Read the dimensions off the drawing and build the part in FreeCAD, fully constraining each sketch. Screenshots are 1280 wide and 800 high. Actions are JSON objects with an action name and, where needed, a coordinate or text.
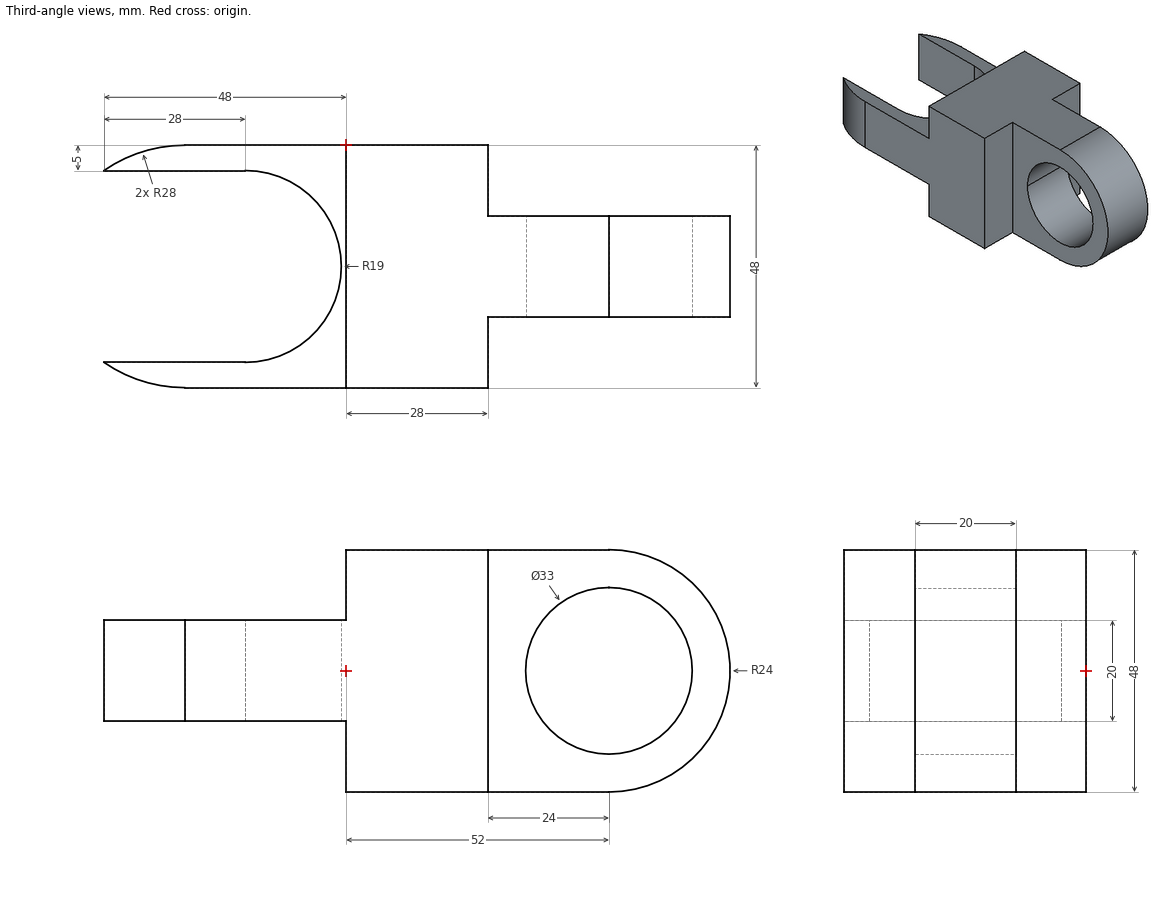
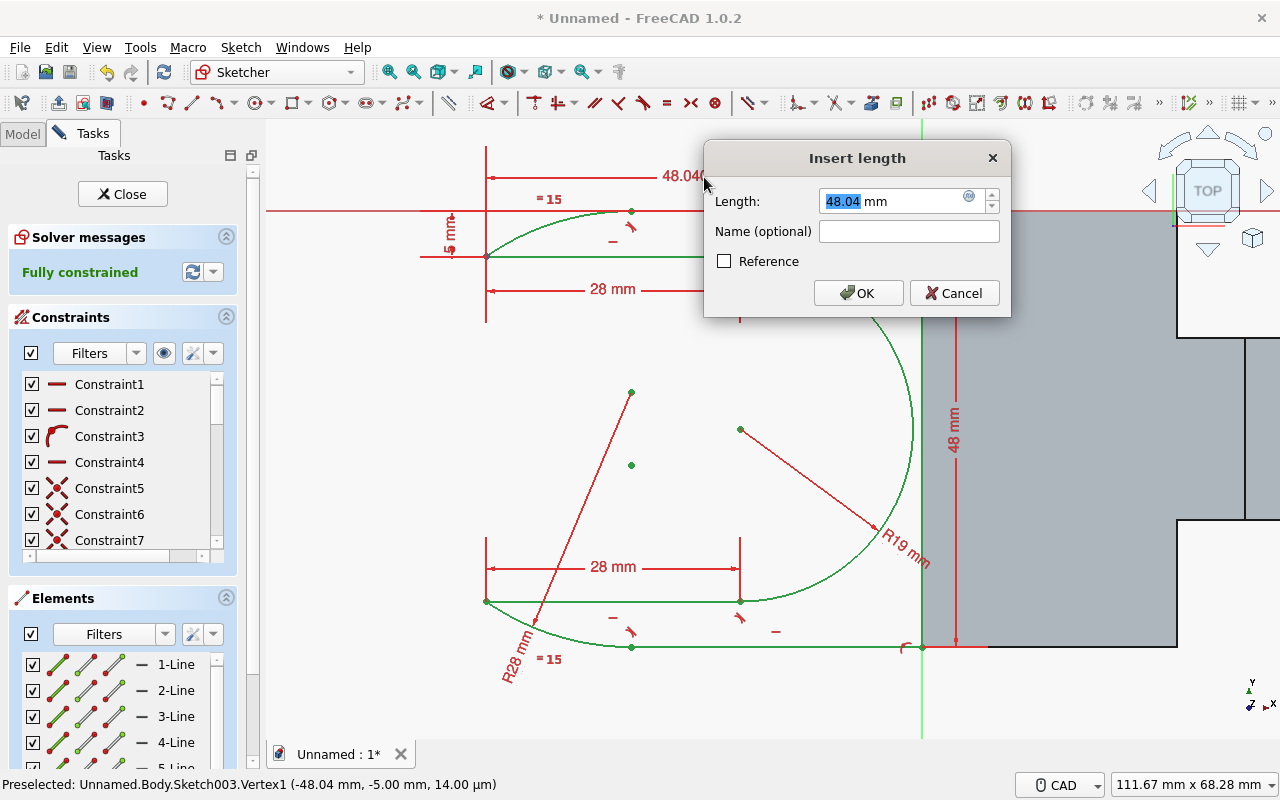
{"action": "type", "text": "48"}
{"action": "key", "text": "Return"}
{"action": "key", "text": "Escape"}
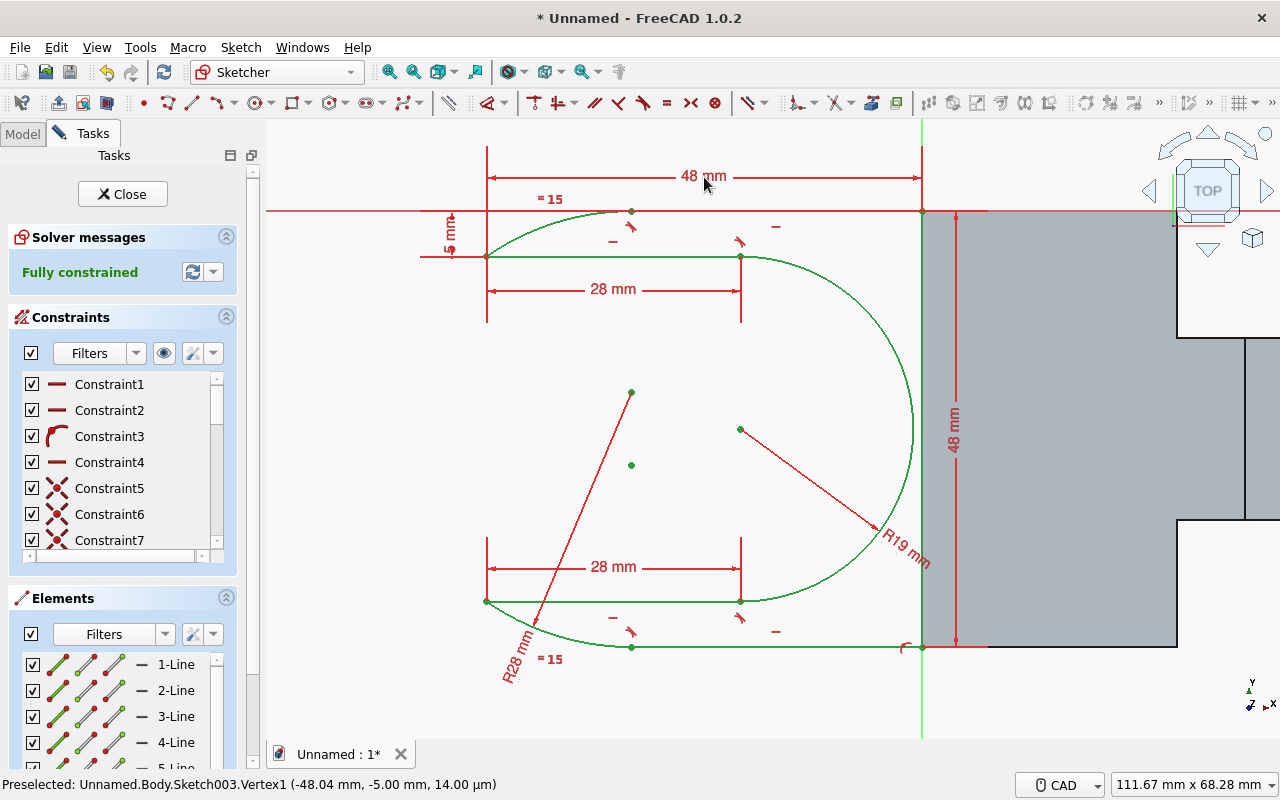
{"action": "left_click", "coordinate": [123, 194]}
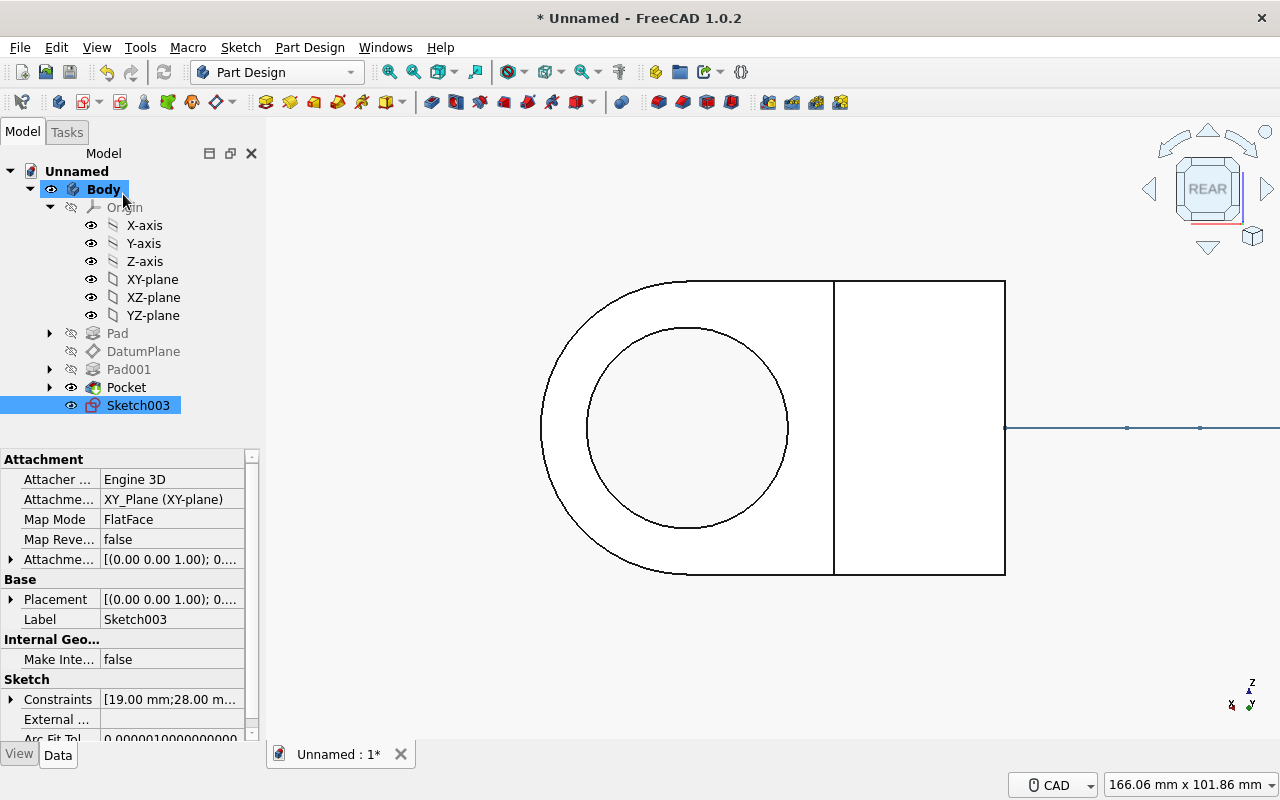
{"action": "left_click", "coordinate": [266, 102]}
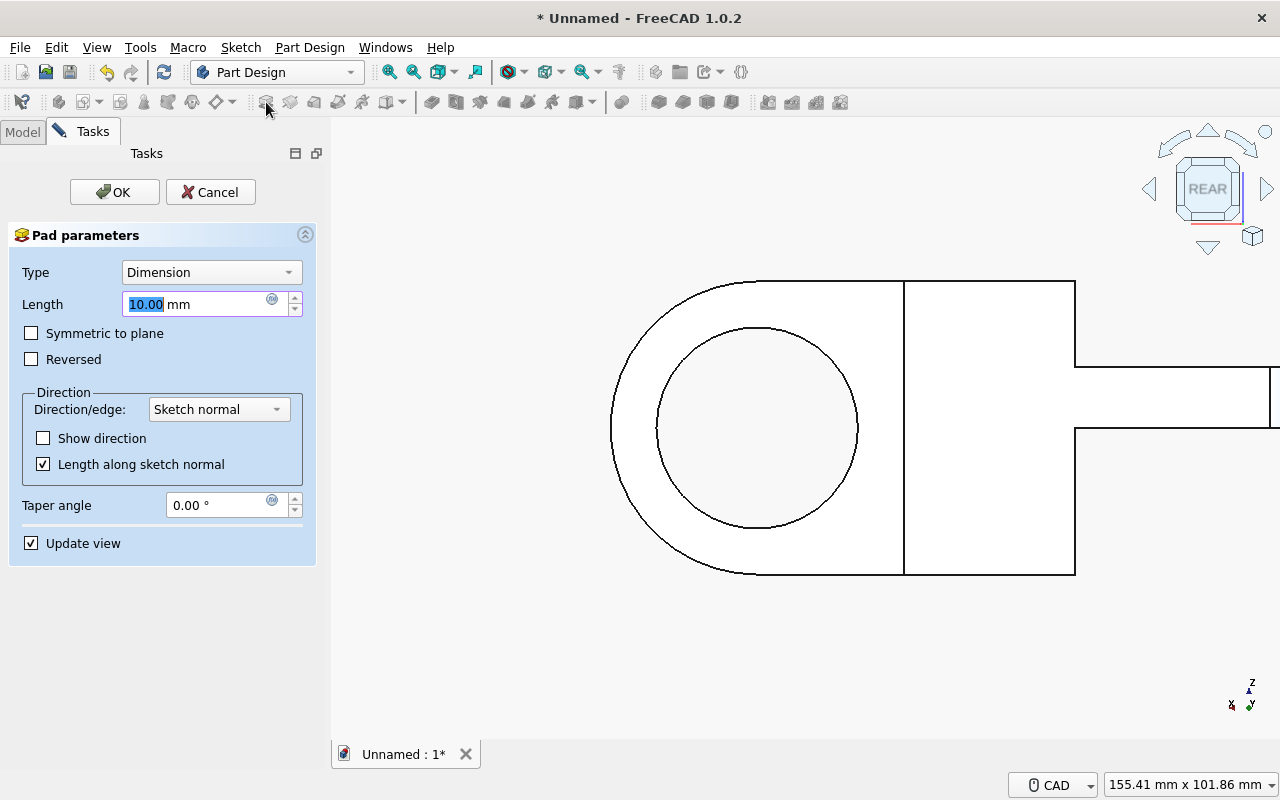
{"action": "type", "text": "20"}
{"action": "key", "text": "Tab"}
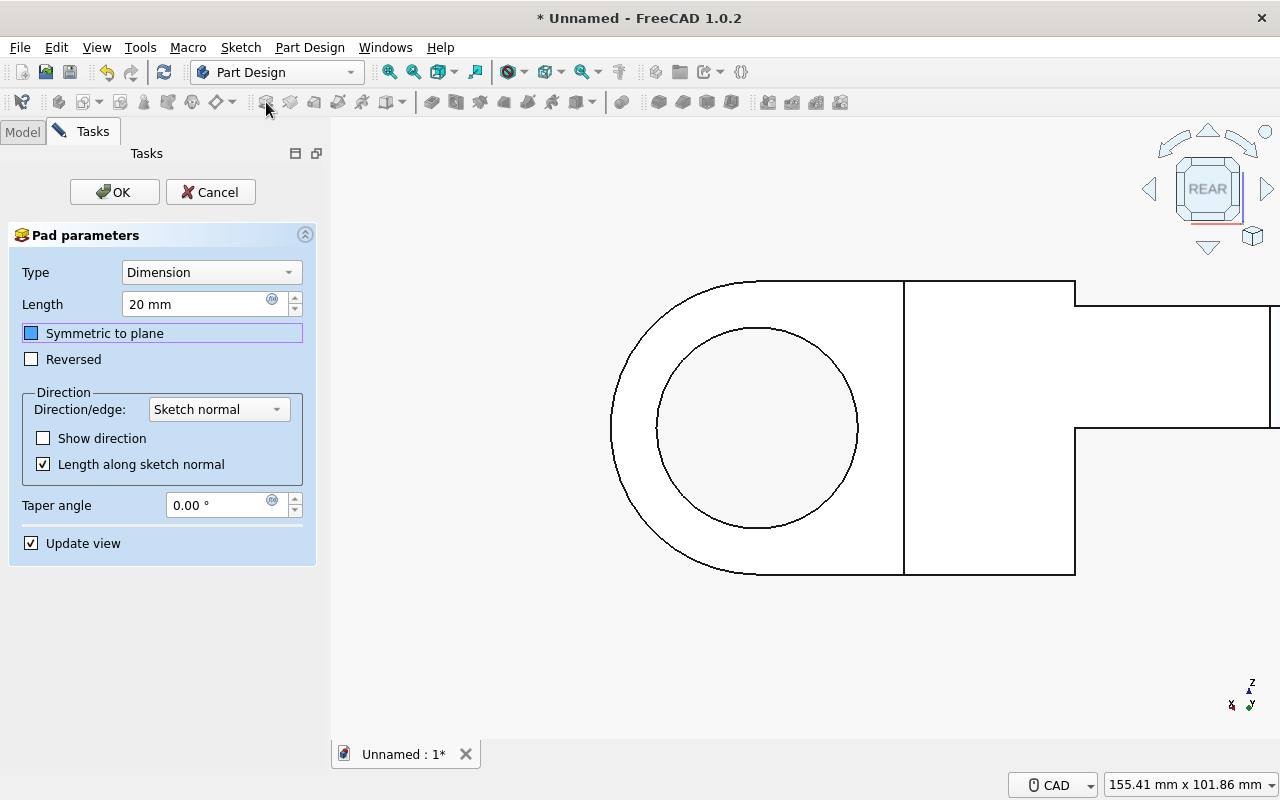
{"action": "left_click", "coordinate": [30, 333]}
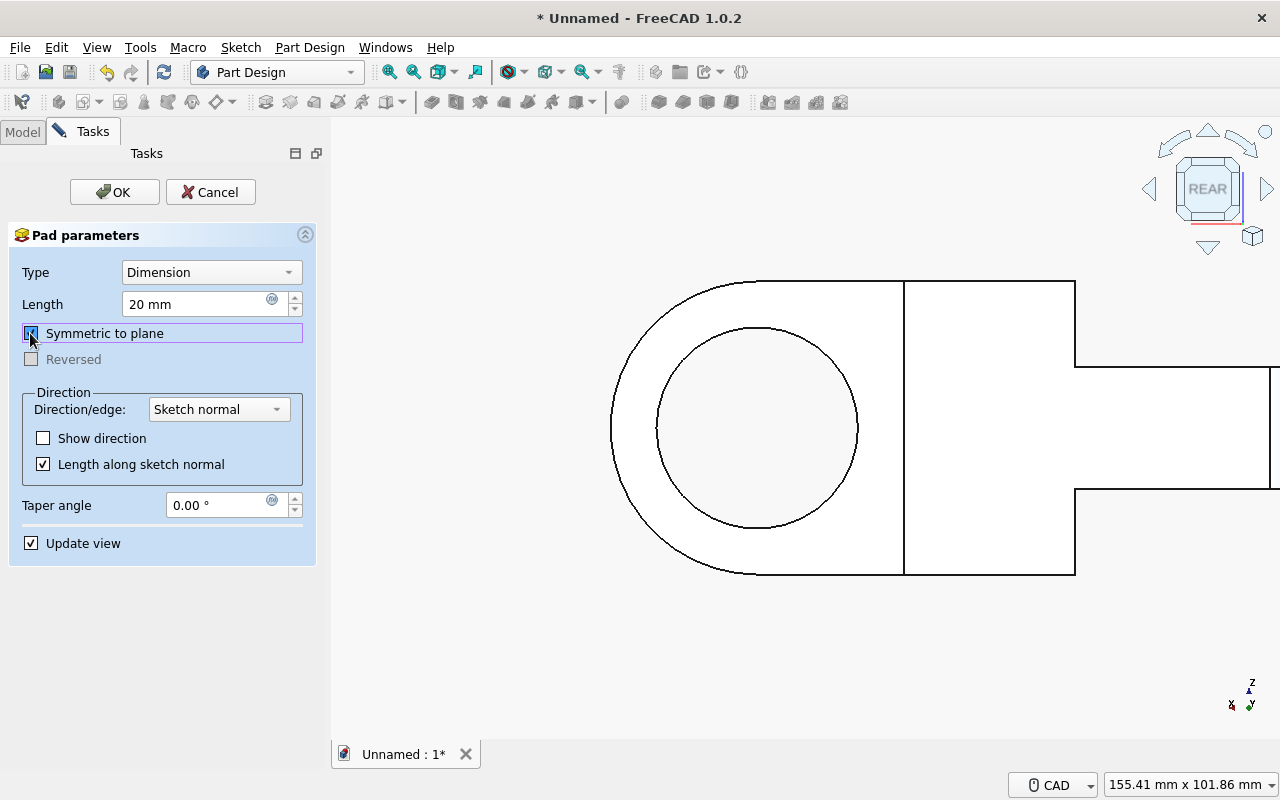
{"action": "left_click", "coordinate": [115, 192]}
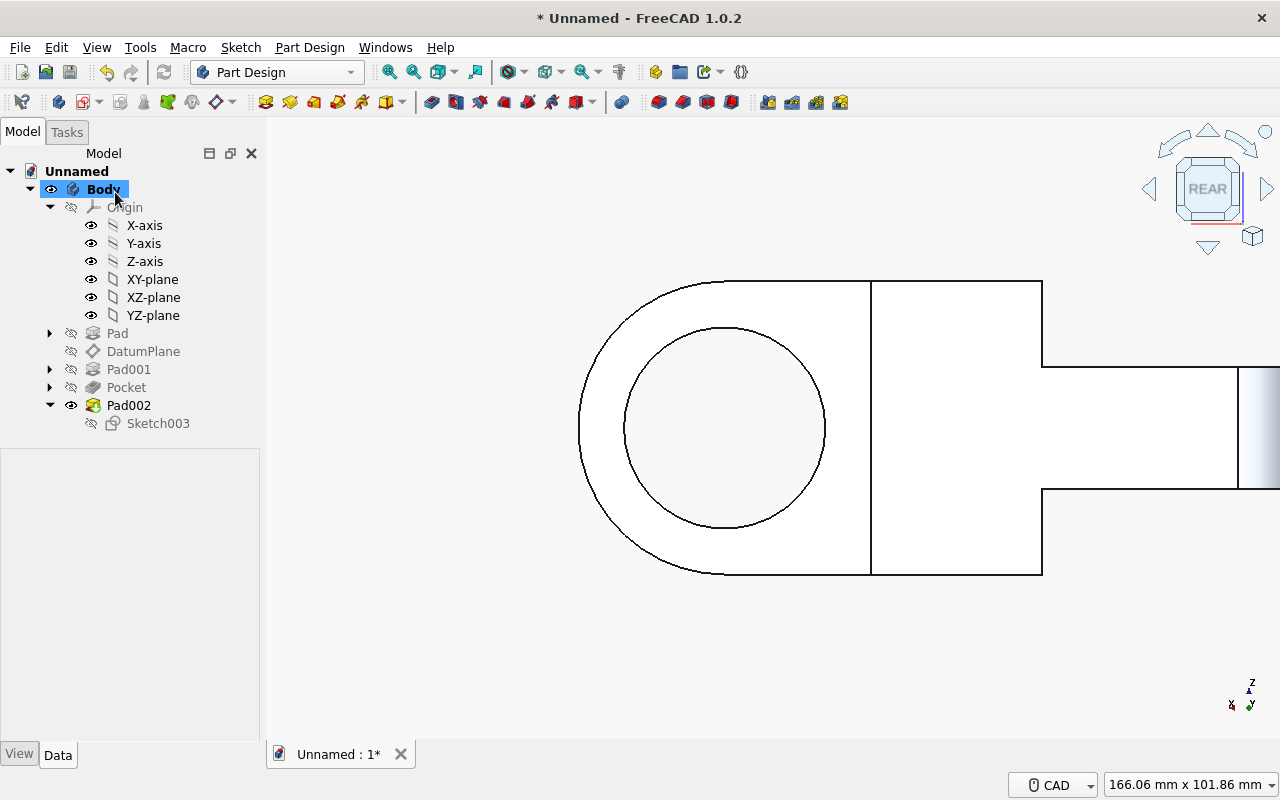
{"action": "key", "text": "0"}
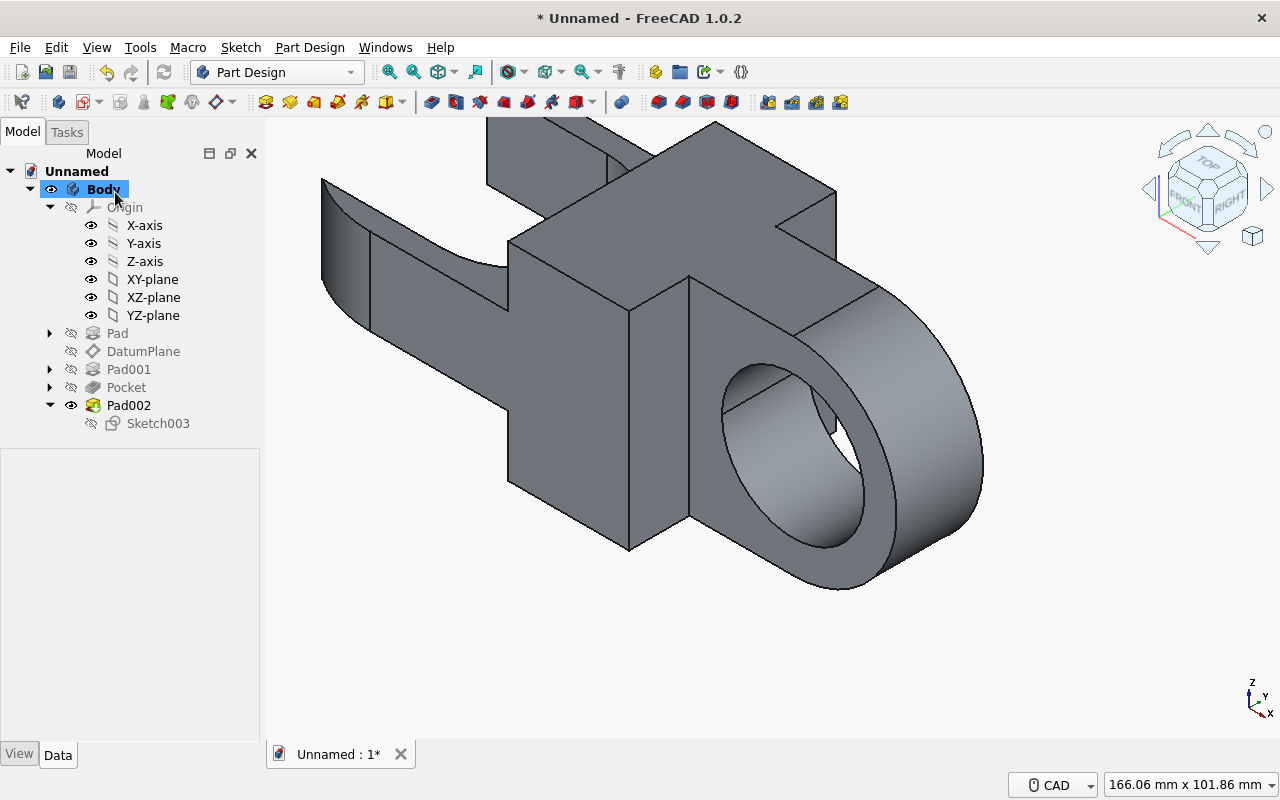
{"action": "left_click", "coordinate": [390, 72]}